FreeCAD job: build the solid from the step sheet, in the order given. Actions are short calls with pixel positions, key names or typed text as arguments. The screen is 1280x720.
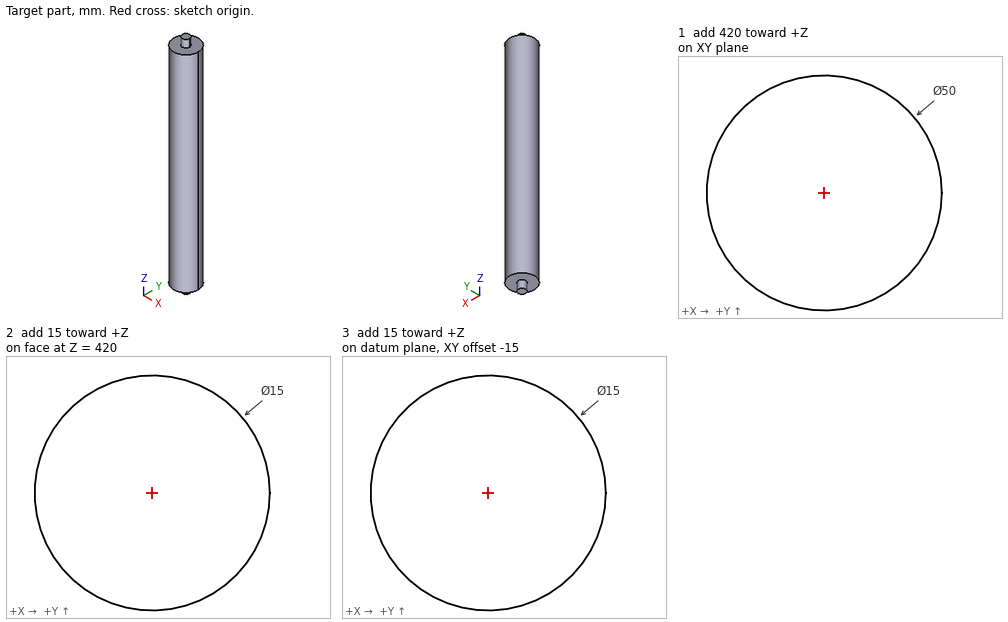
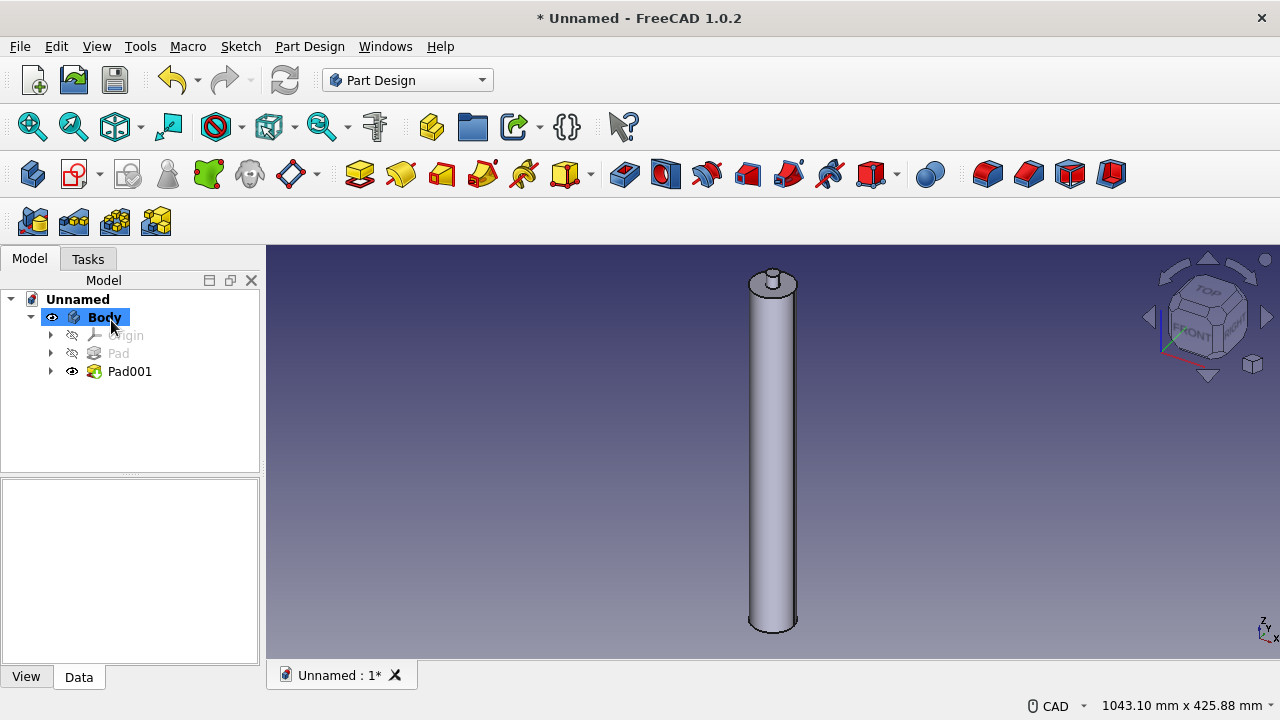
click(51, 335)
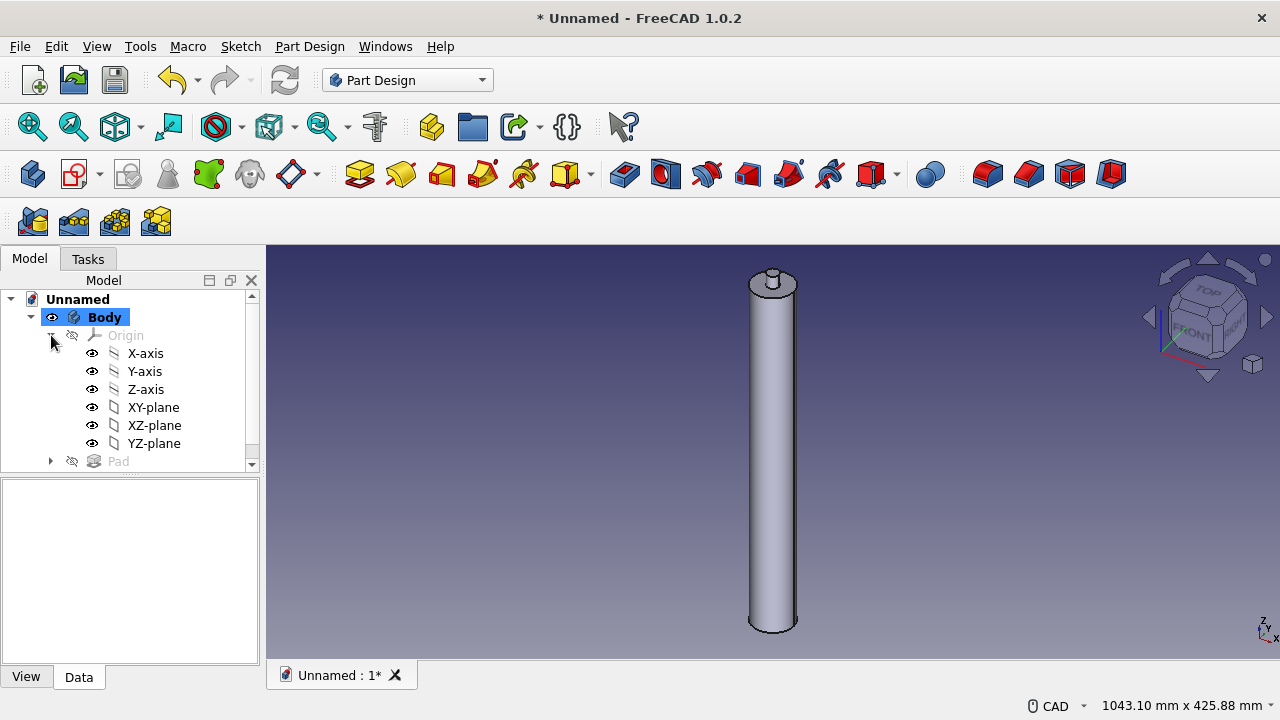
click(137, 407)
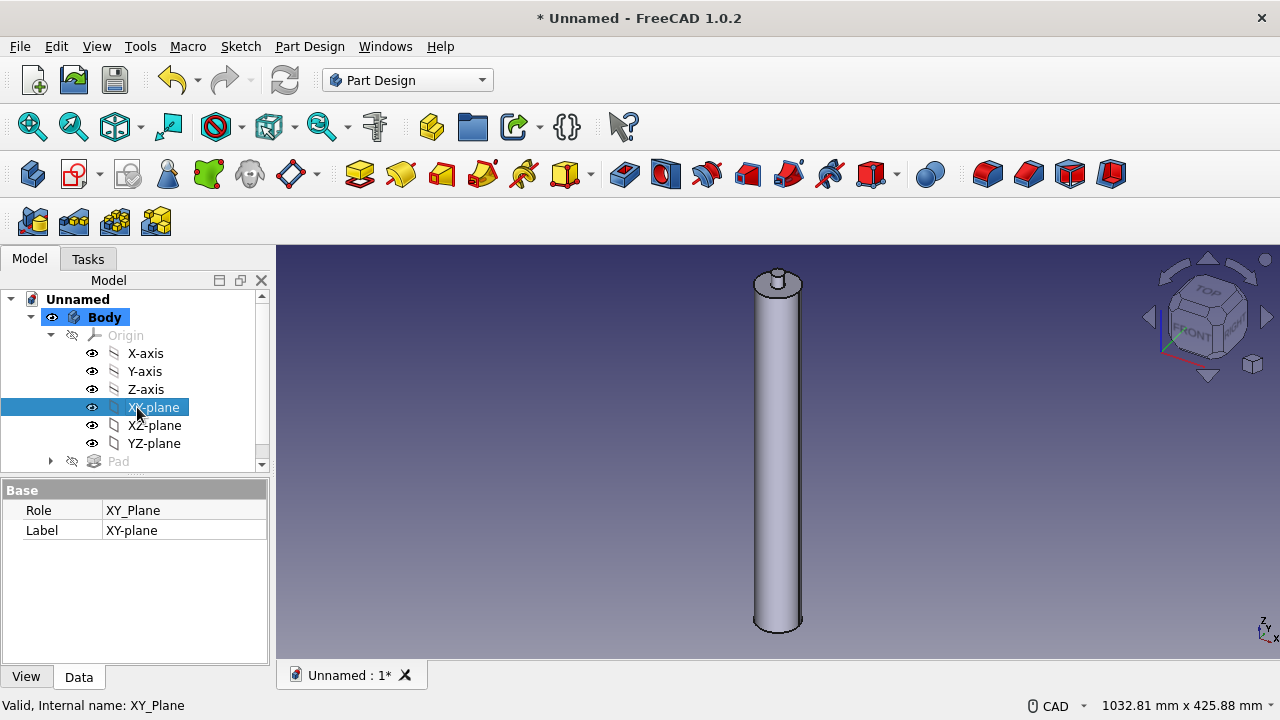
click(290, 174)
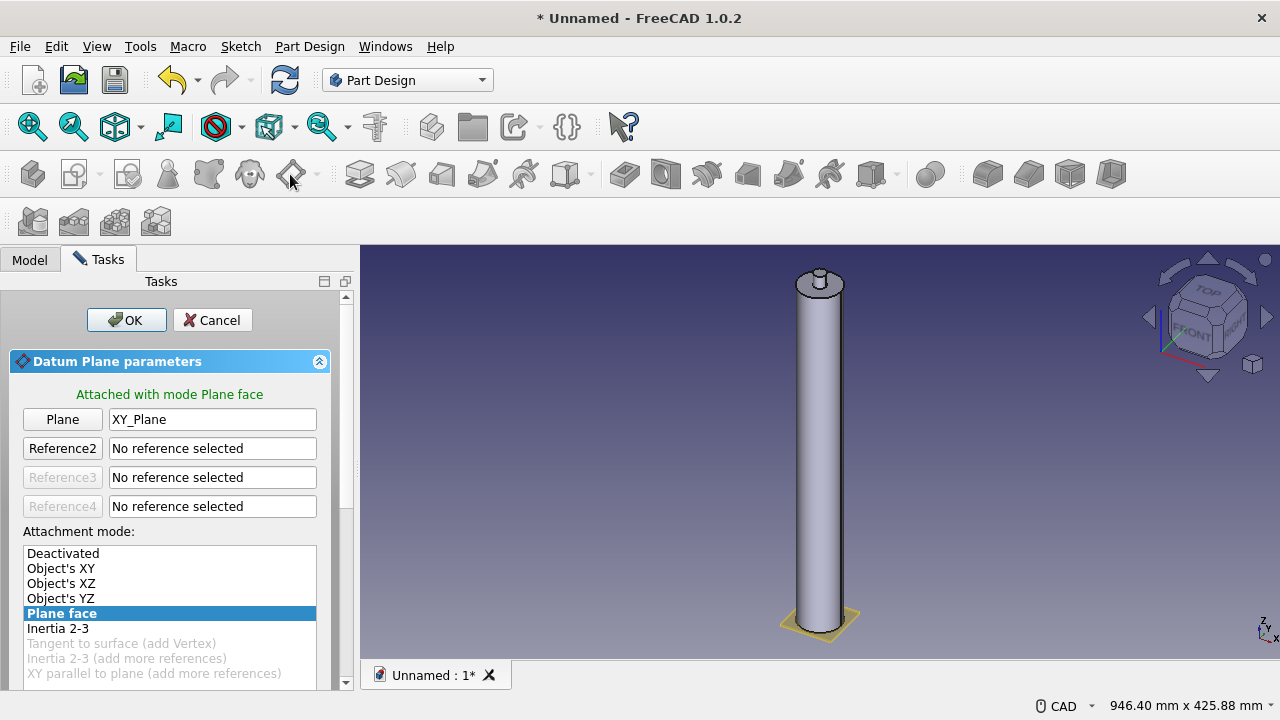
scroll(346, 490, down, 4)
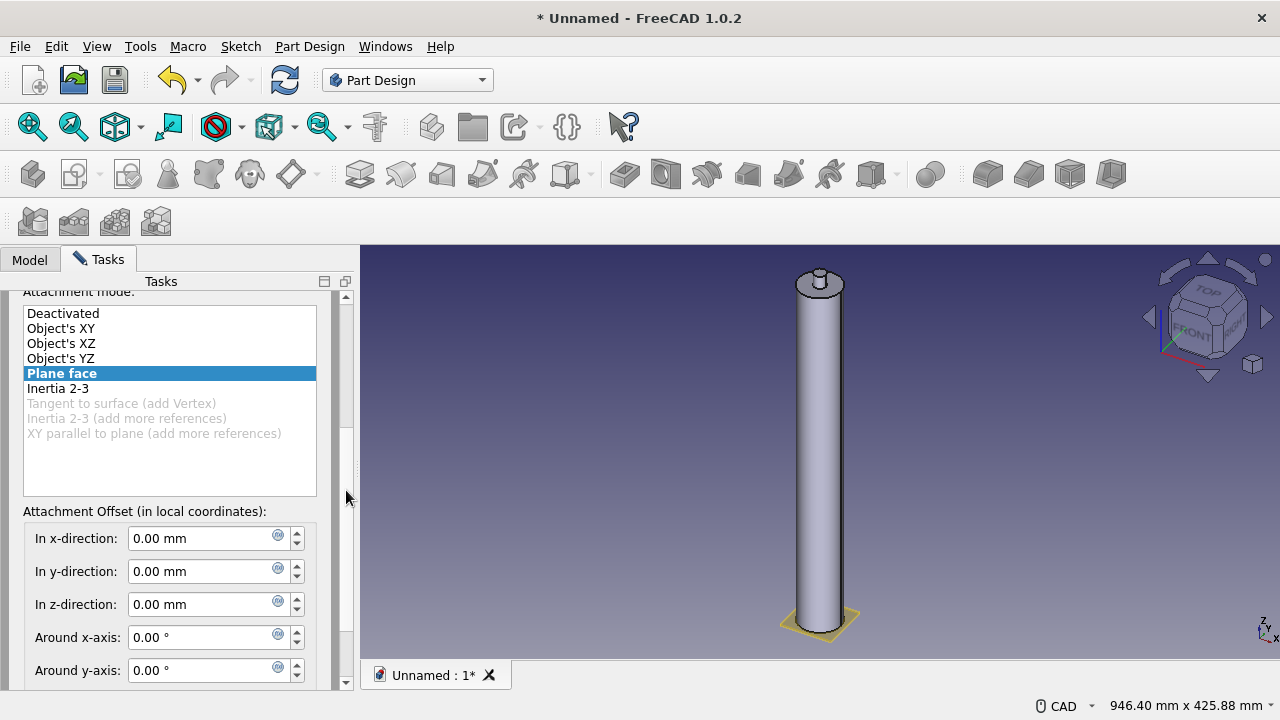
triple_click(210, 604)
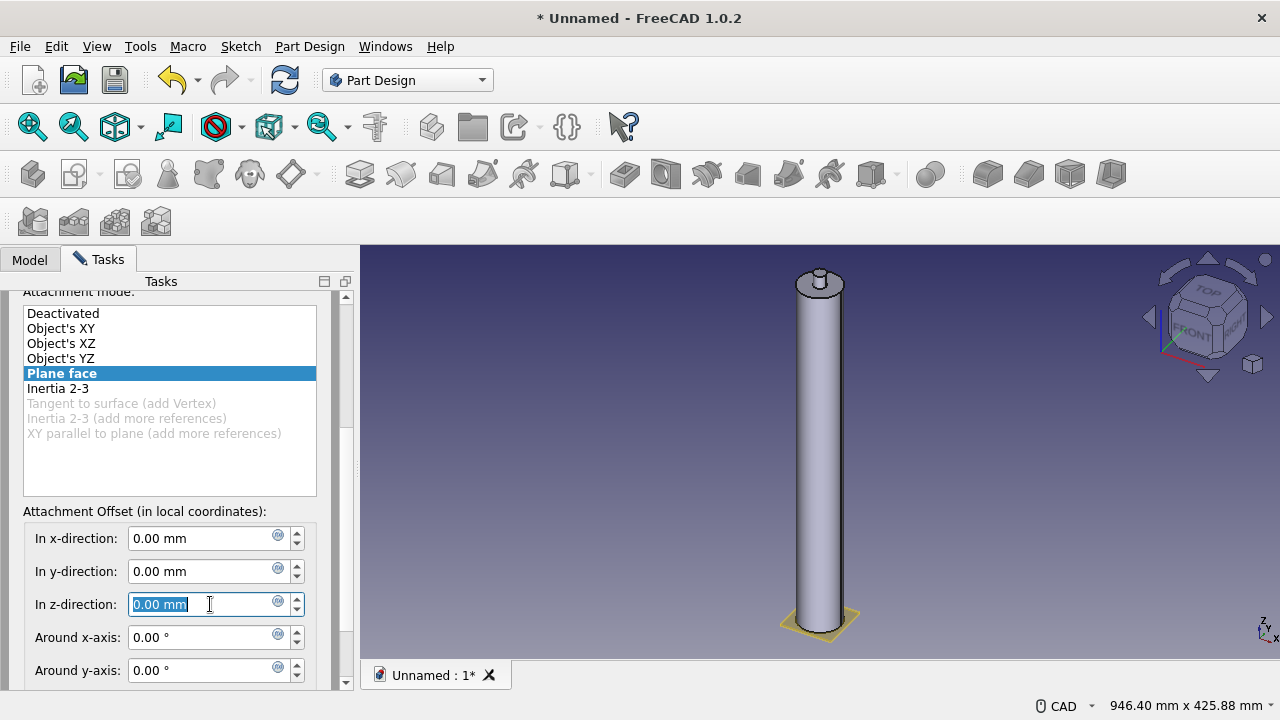
text(-15)
key(Tab)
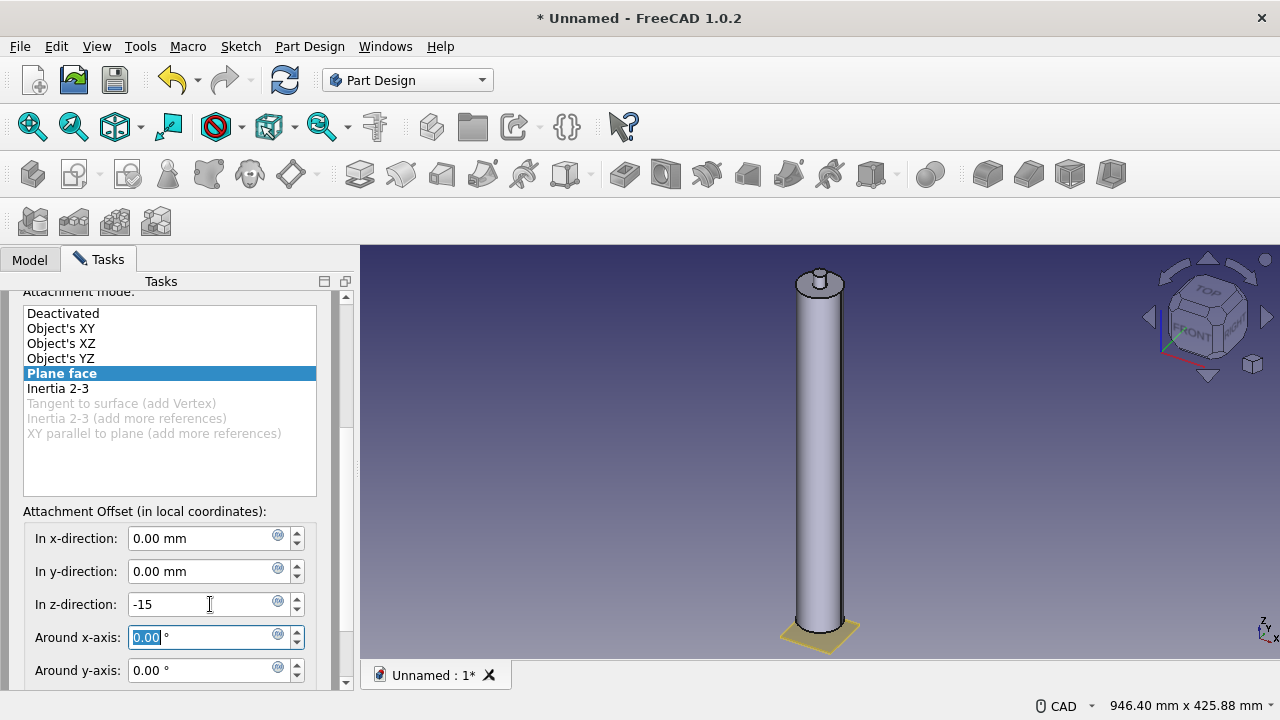
scroll(346, 490, up, 5)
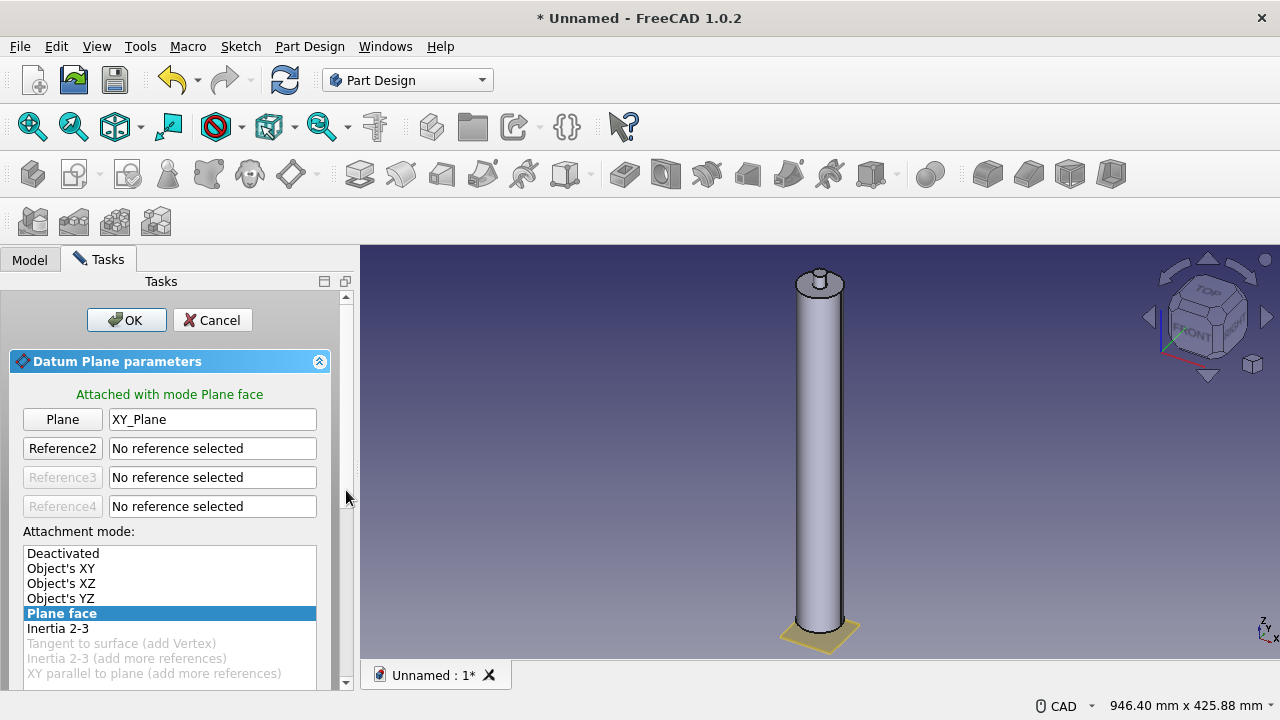
click(127, 320)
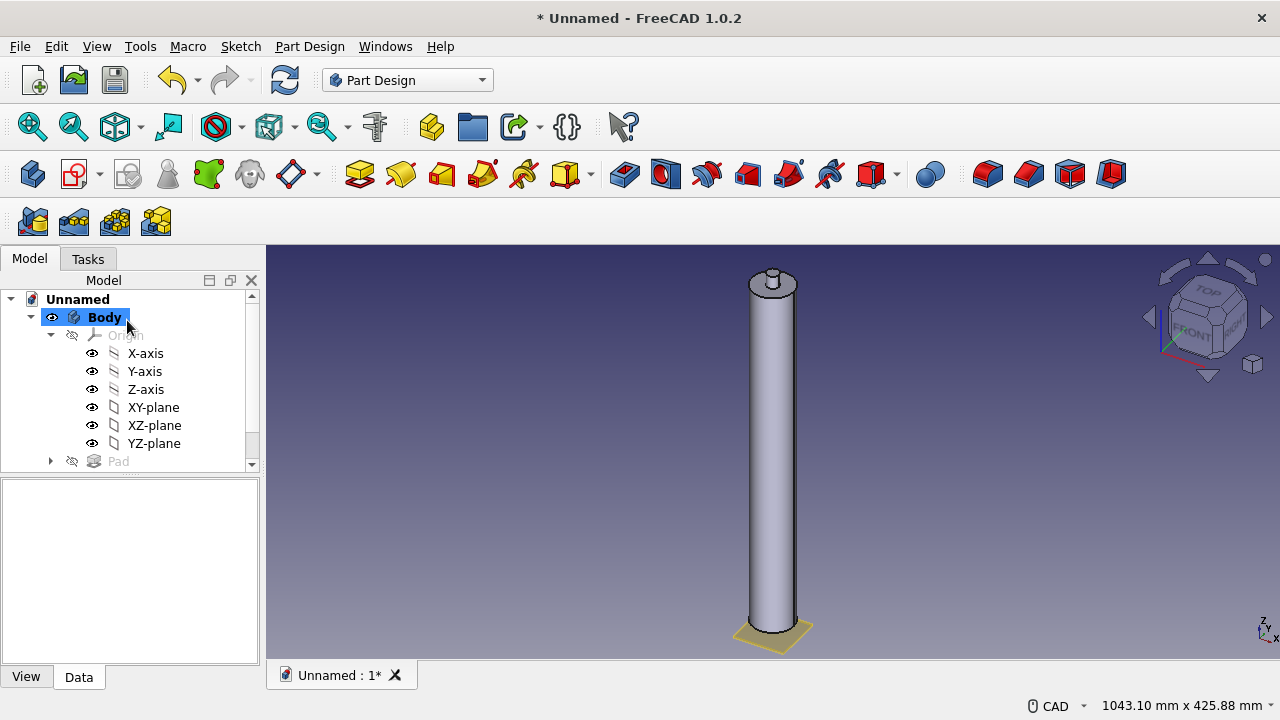
scroll(101, 385, down, 3)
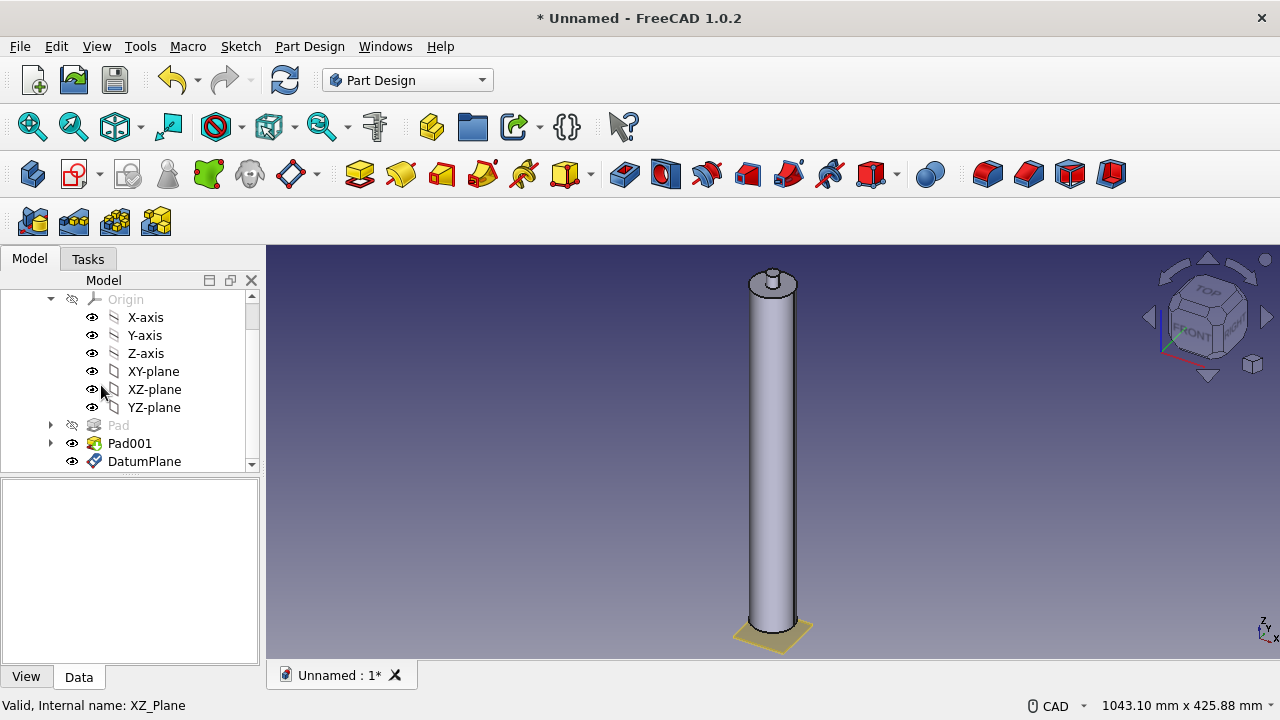
click(117, 461)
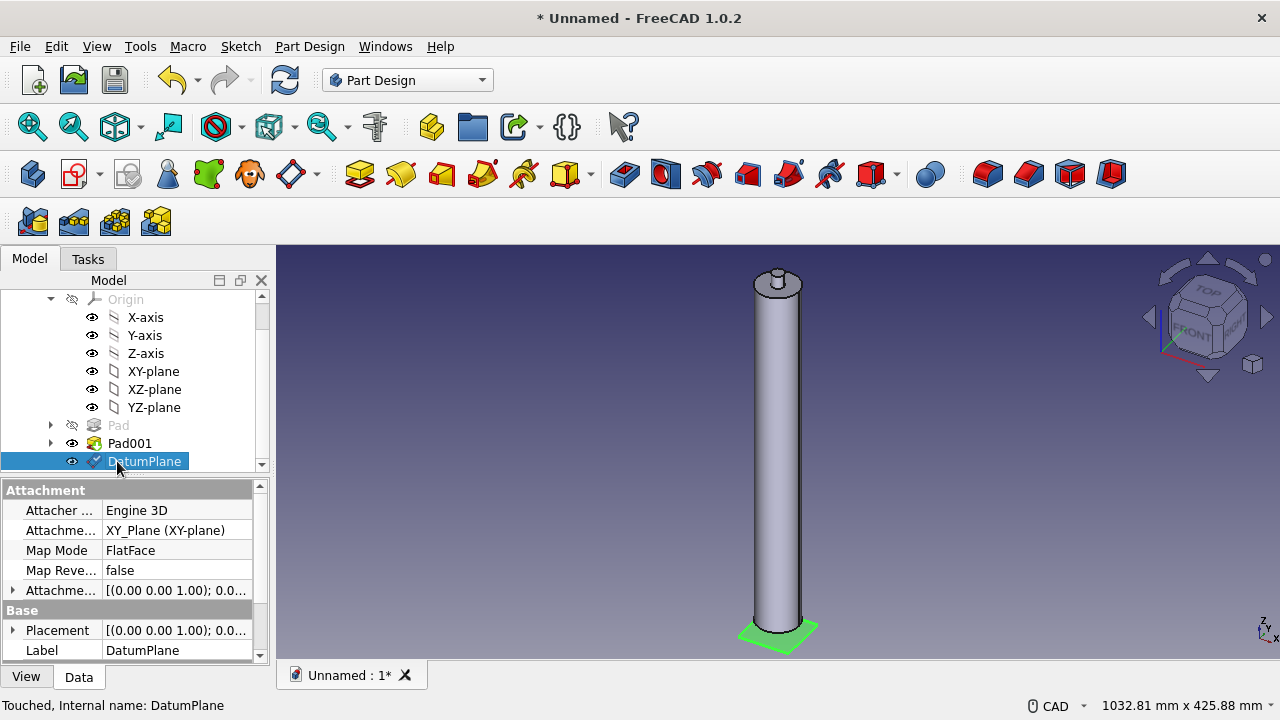
click(74, 174)